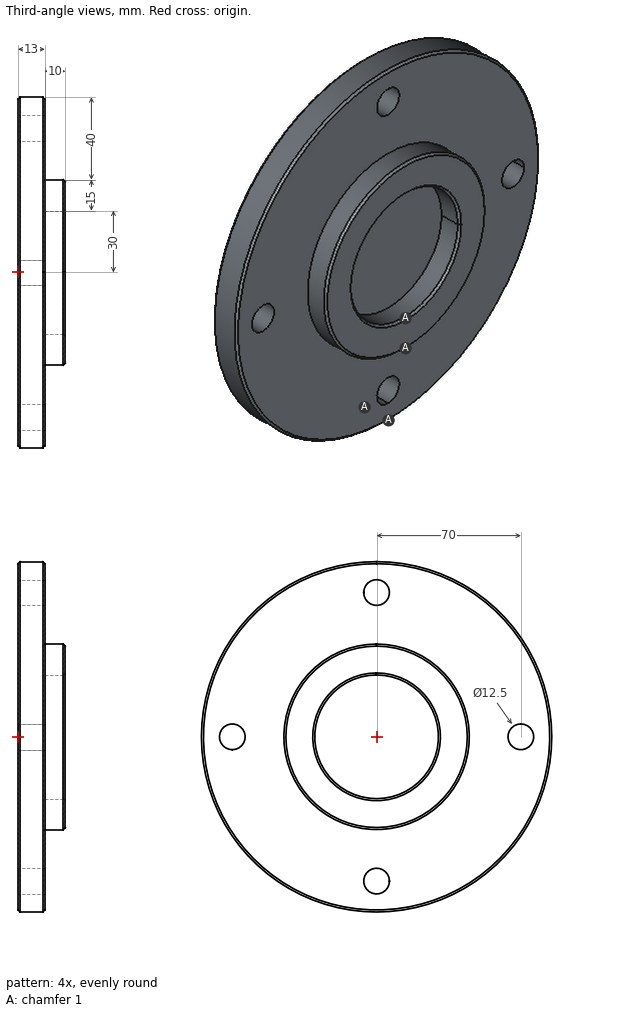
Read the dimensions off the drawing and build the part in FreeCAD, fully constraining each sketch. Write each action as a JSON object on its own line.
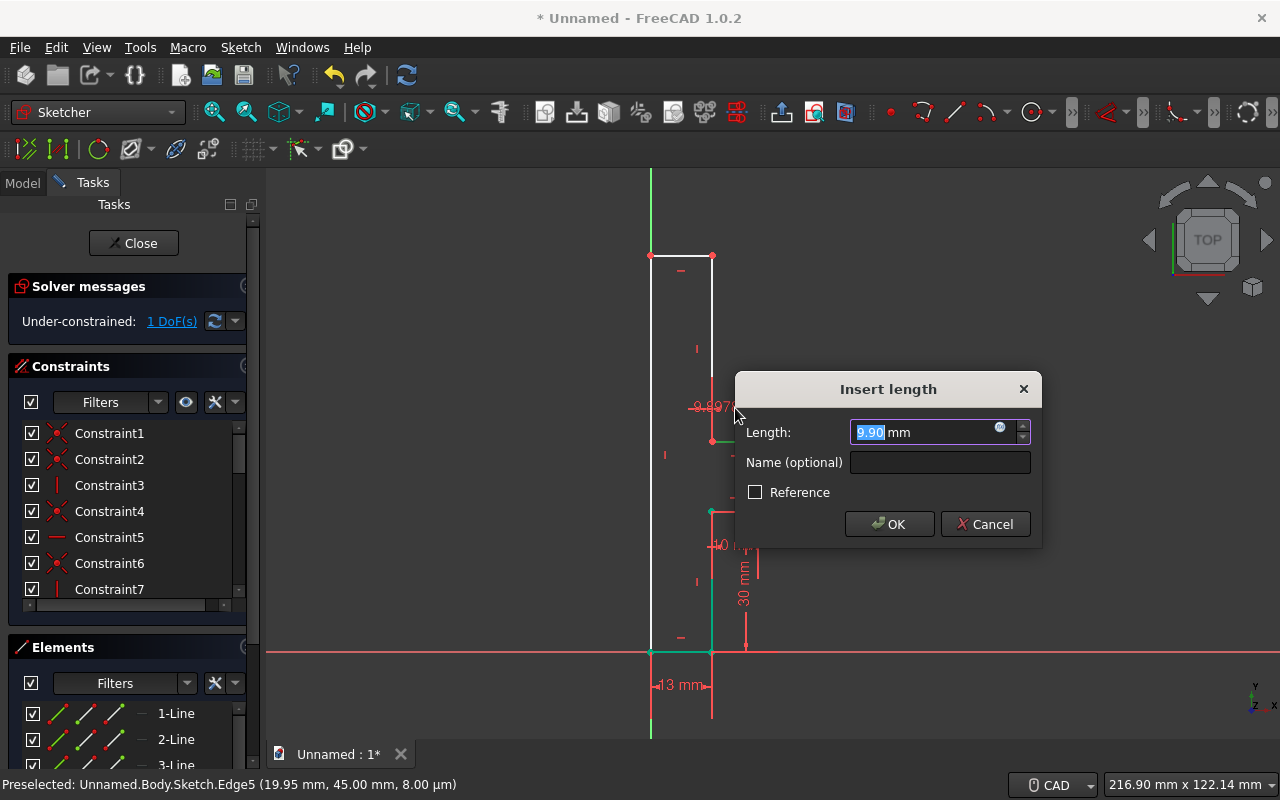
{"action": "type", "text": "10"}
{"action": "key", "text": "Return"}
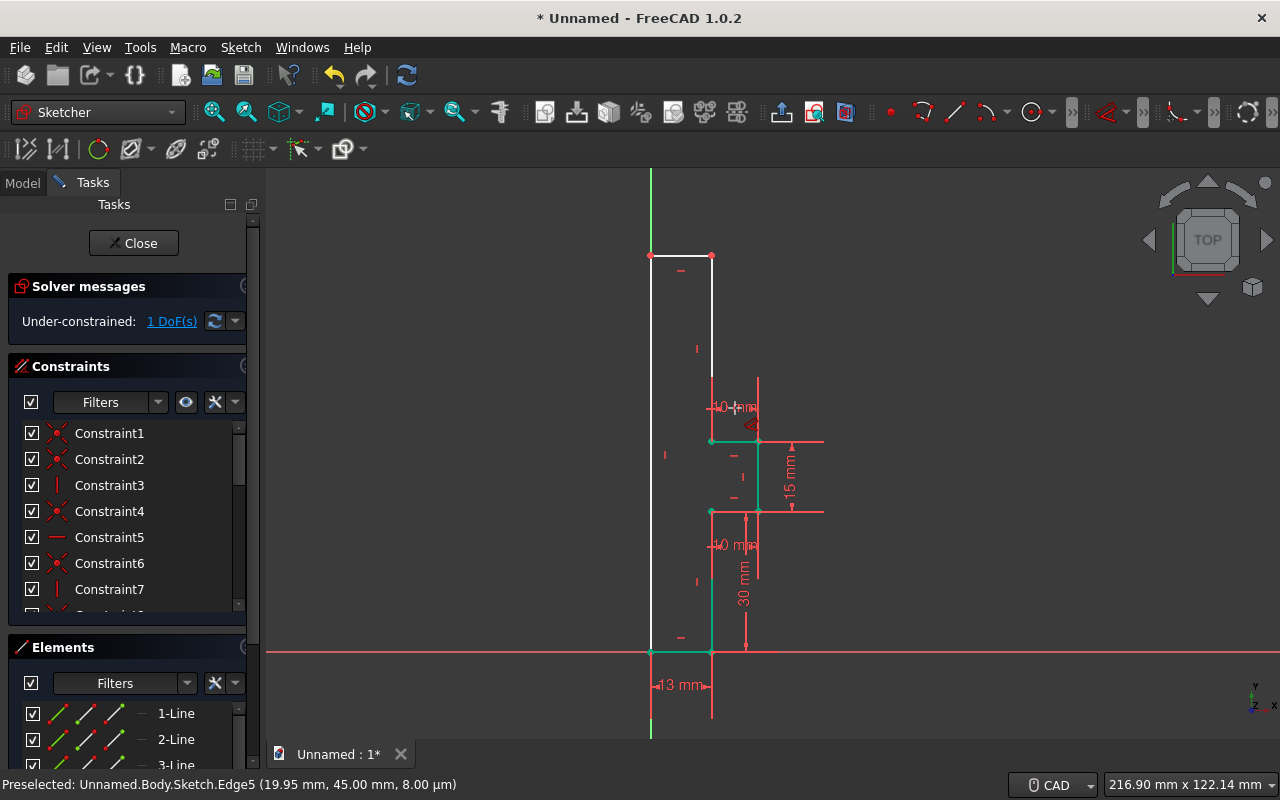
{"action": "left_click", "coordinate": [712, 386]}
{"action": "left_click", "coordinate": [746, 349]}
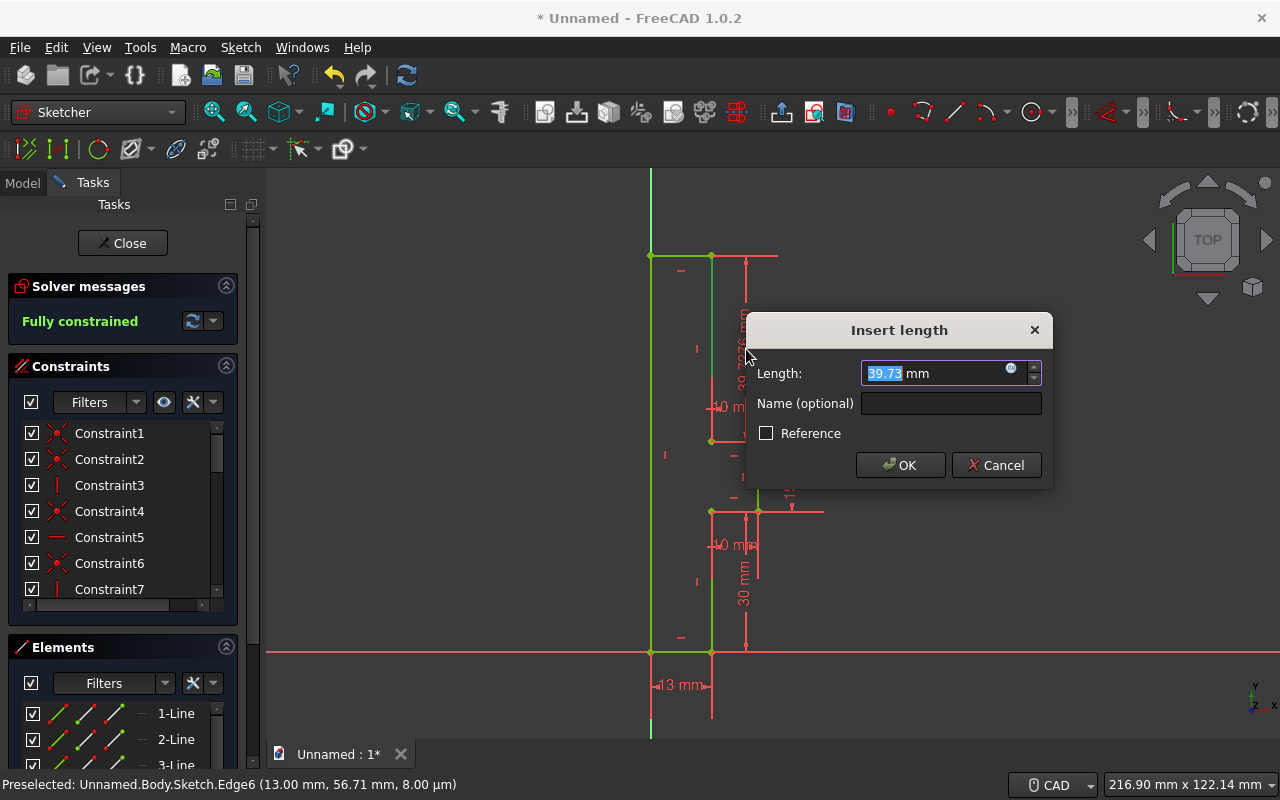
{"action": "type", "text": "40"}
{"action": "key", "text": "Return"}
{"action": "key", "text": "Escape"}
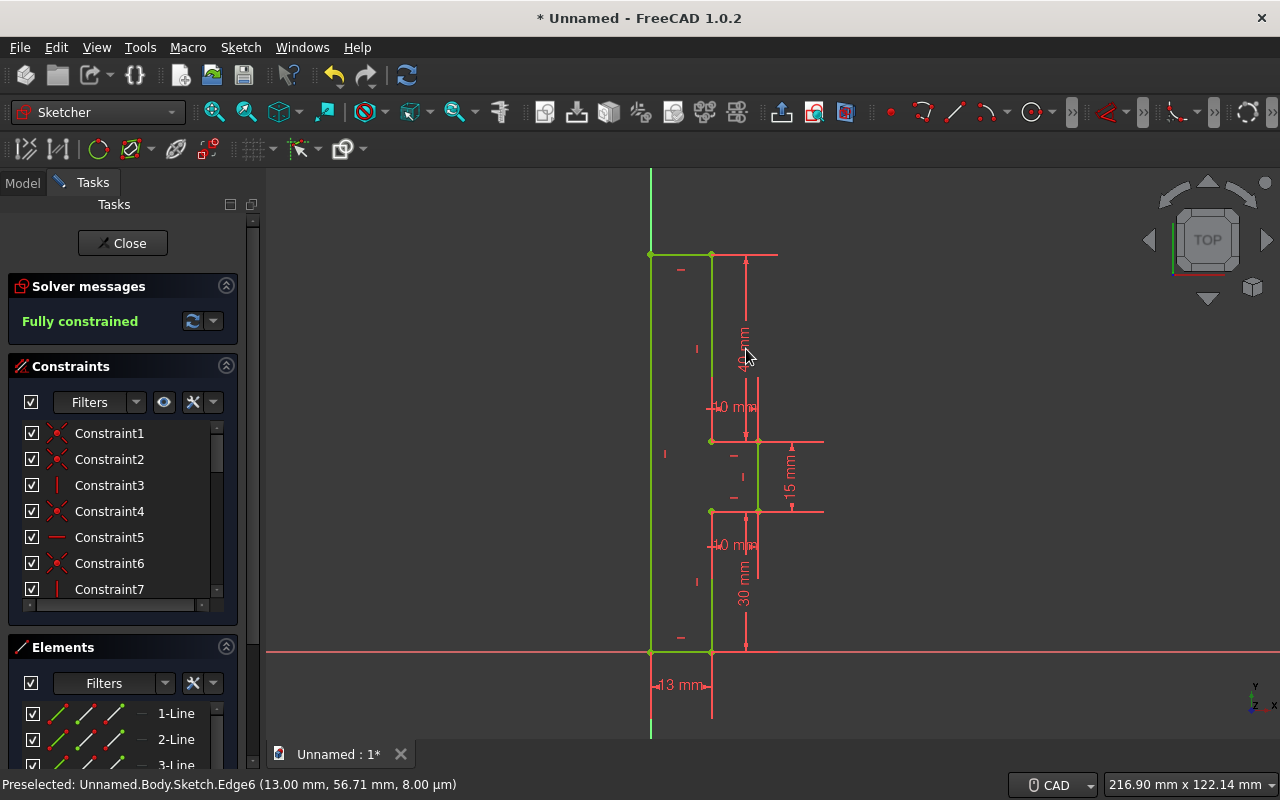
{"action": "left_click", "coordinate": [123, 243]}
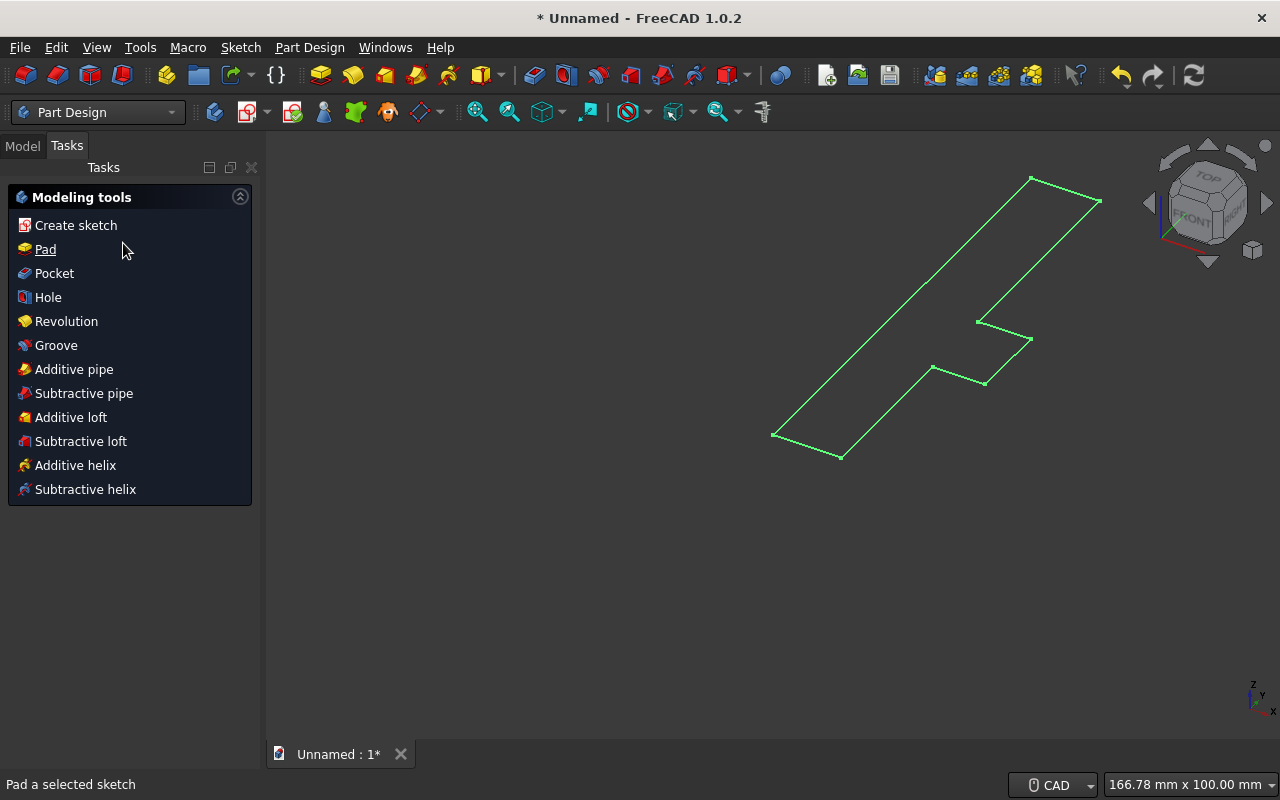
{"action": "left_click", "coordinate": [354, 76]}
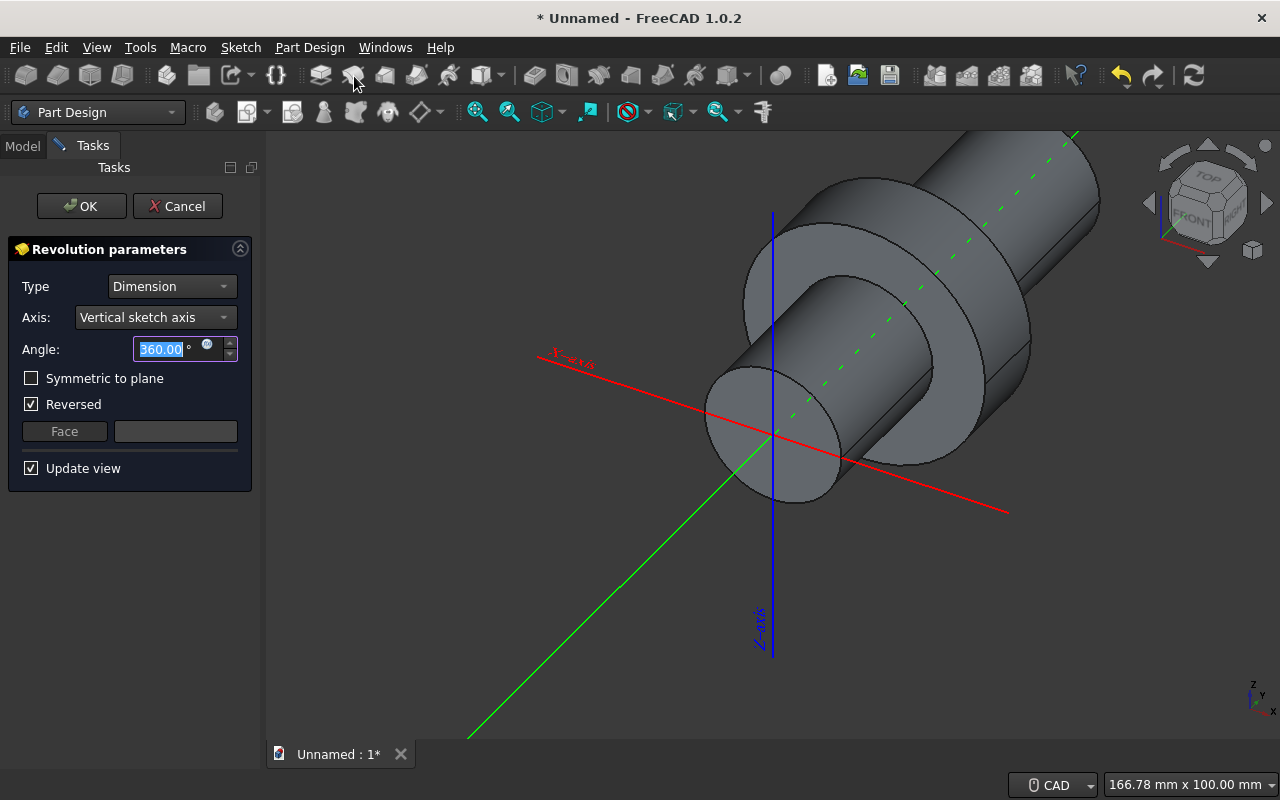
{"action": "left_click", "coordinate": [156, 318]}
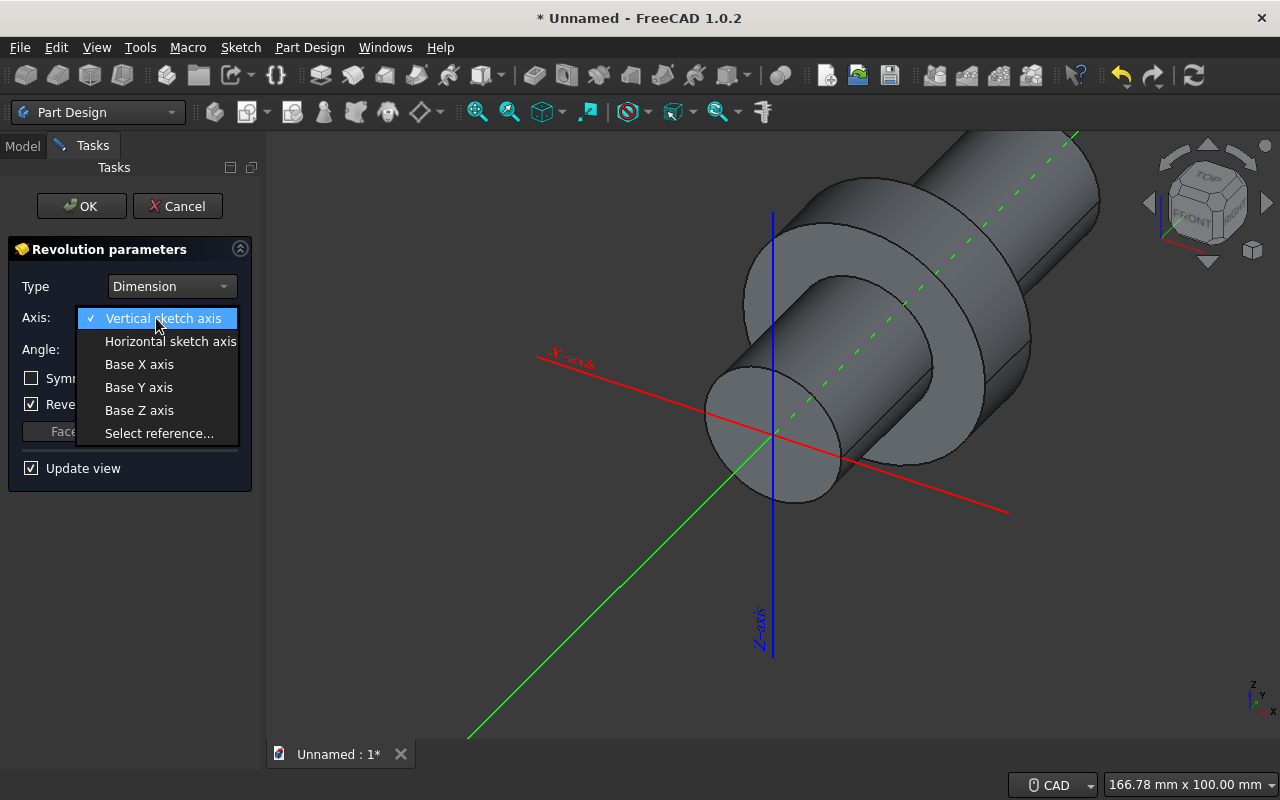
{"action": "left_click", "coordinate": [156, 342]}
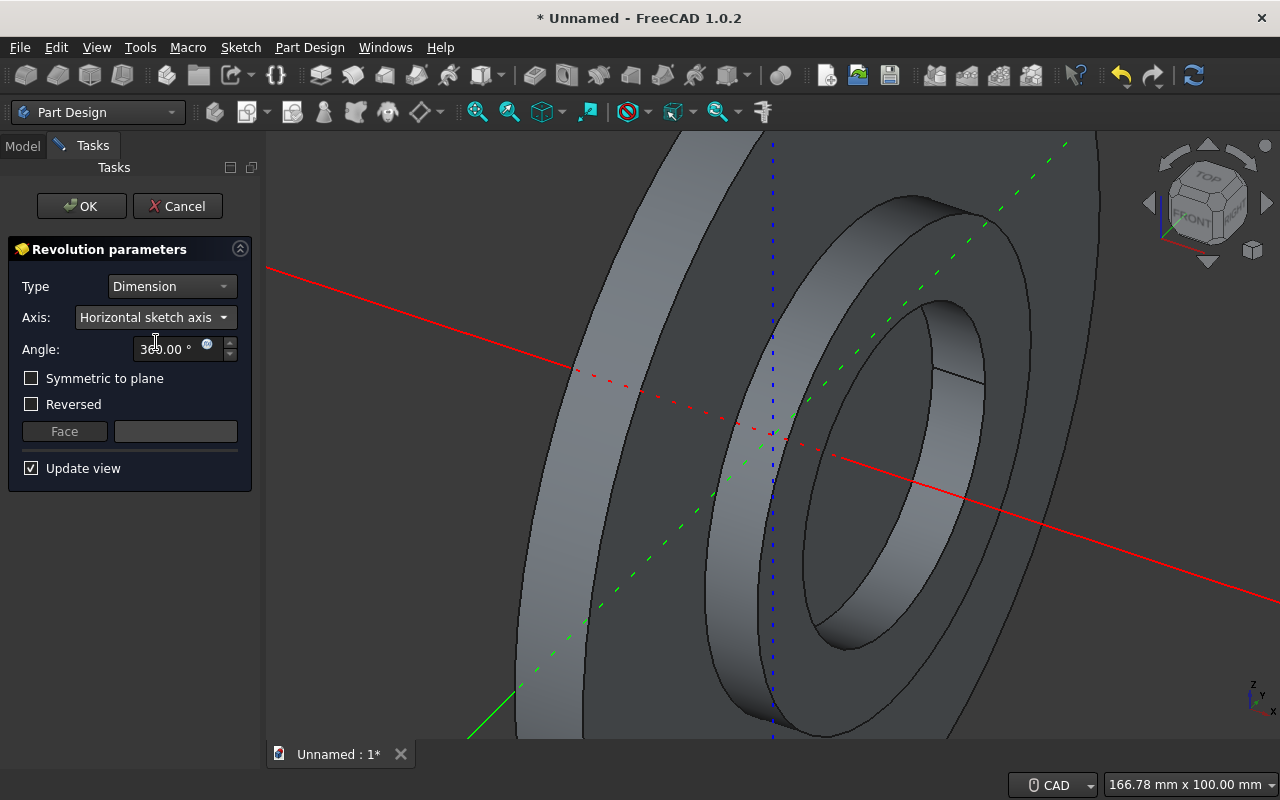
{"action": "left_click", "coordinate": [82, 206]}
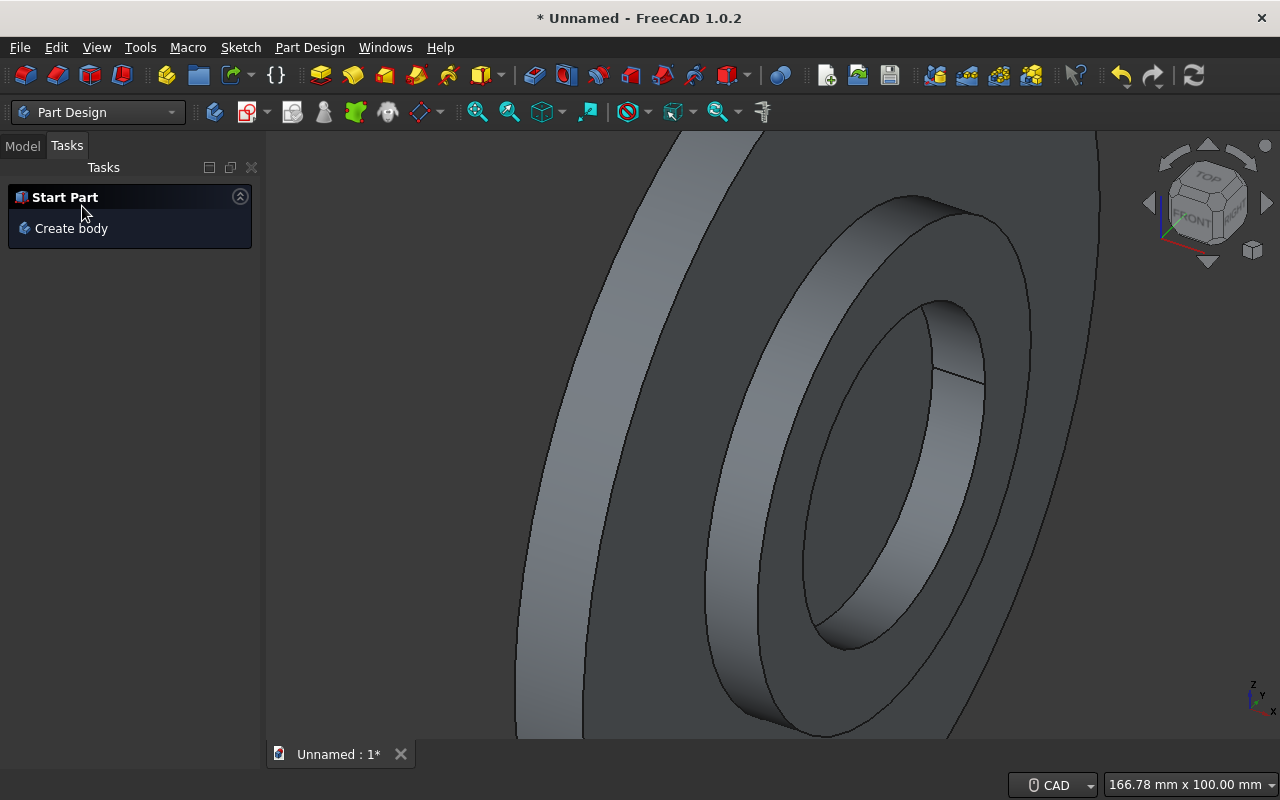
{"action": "key", "text": "v f"}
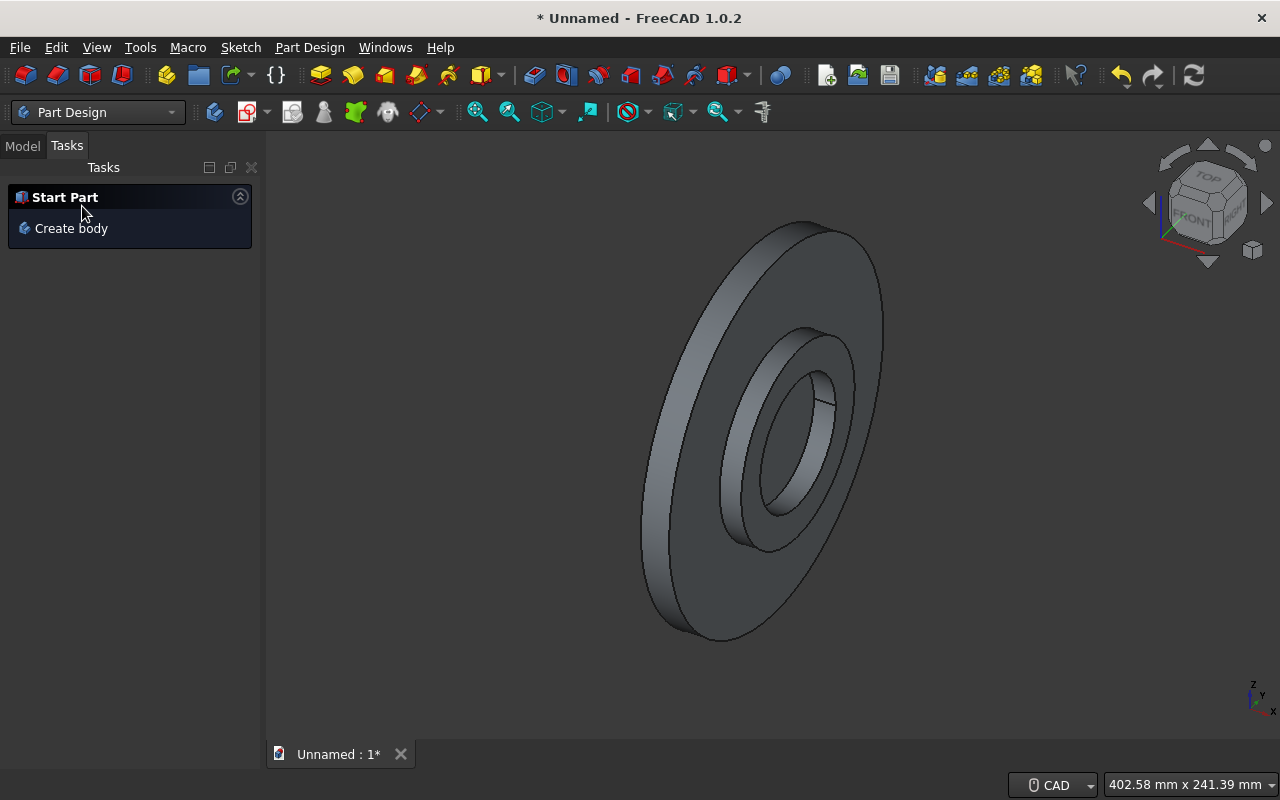
{"action": "left_click", "coordinate": [248, 112]}